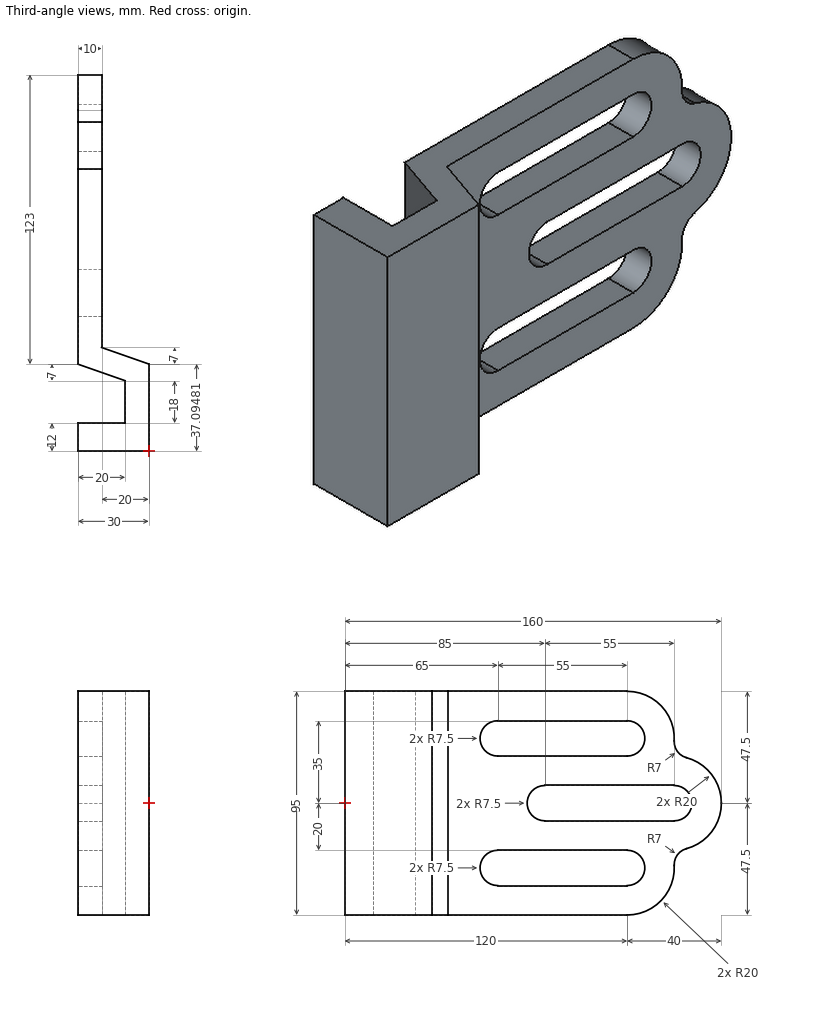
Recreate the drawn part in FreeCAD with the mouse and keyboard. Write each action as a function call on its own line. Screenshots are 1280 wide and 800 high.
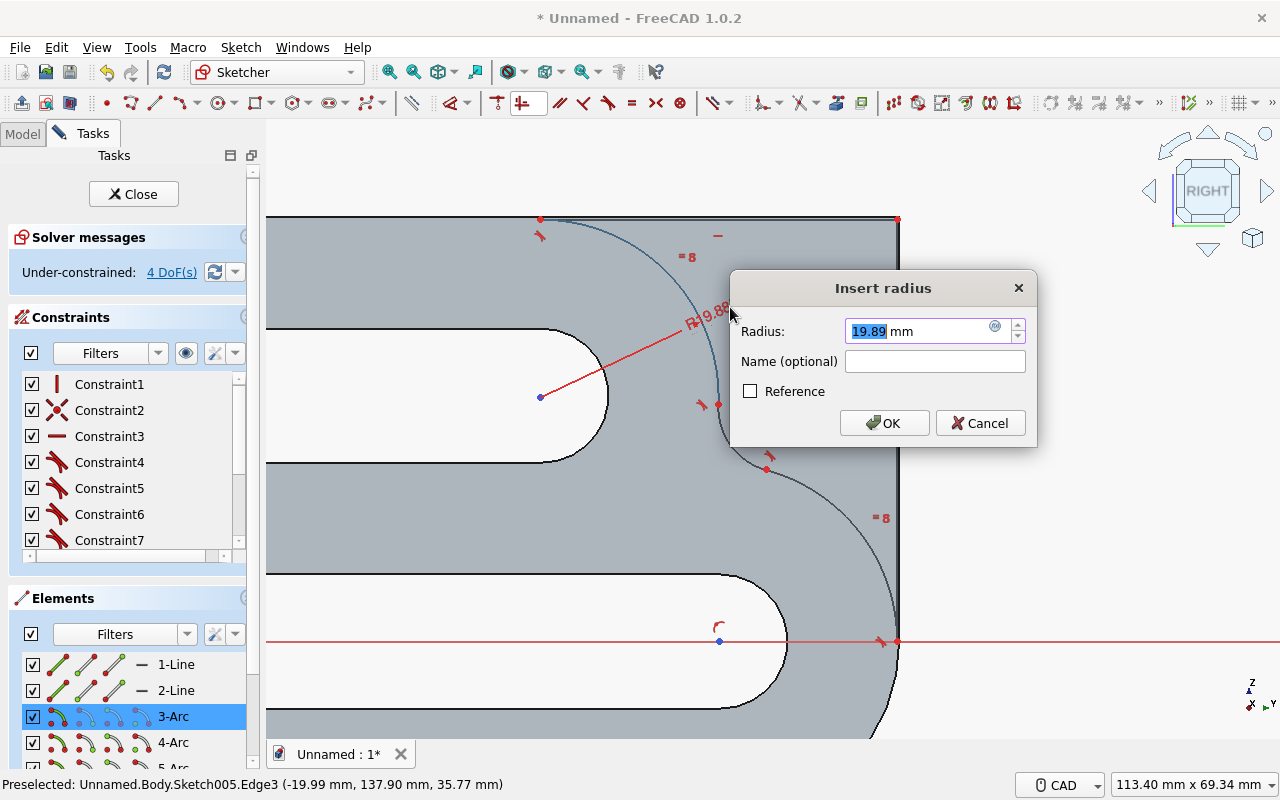
text(20)
key(Return)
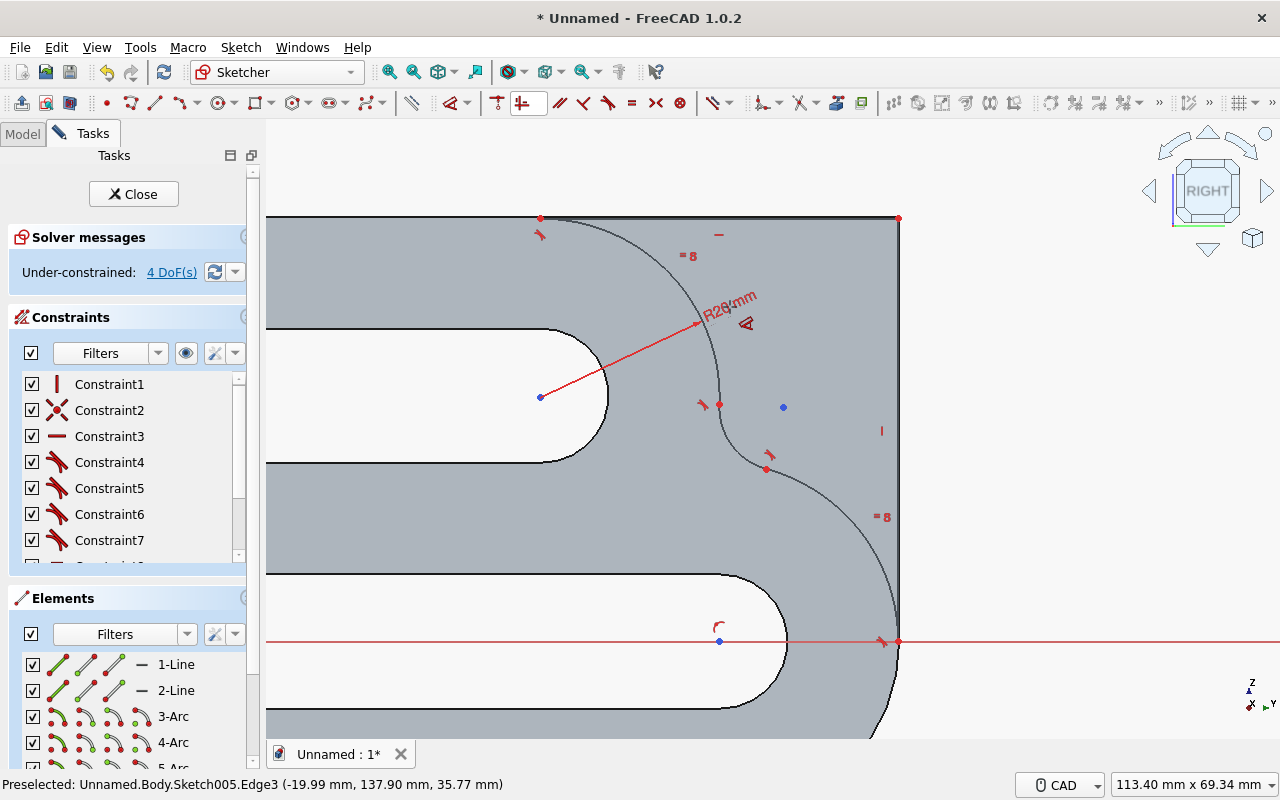
click(724, 430)
click(694, 441)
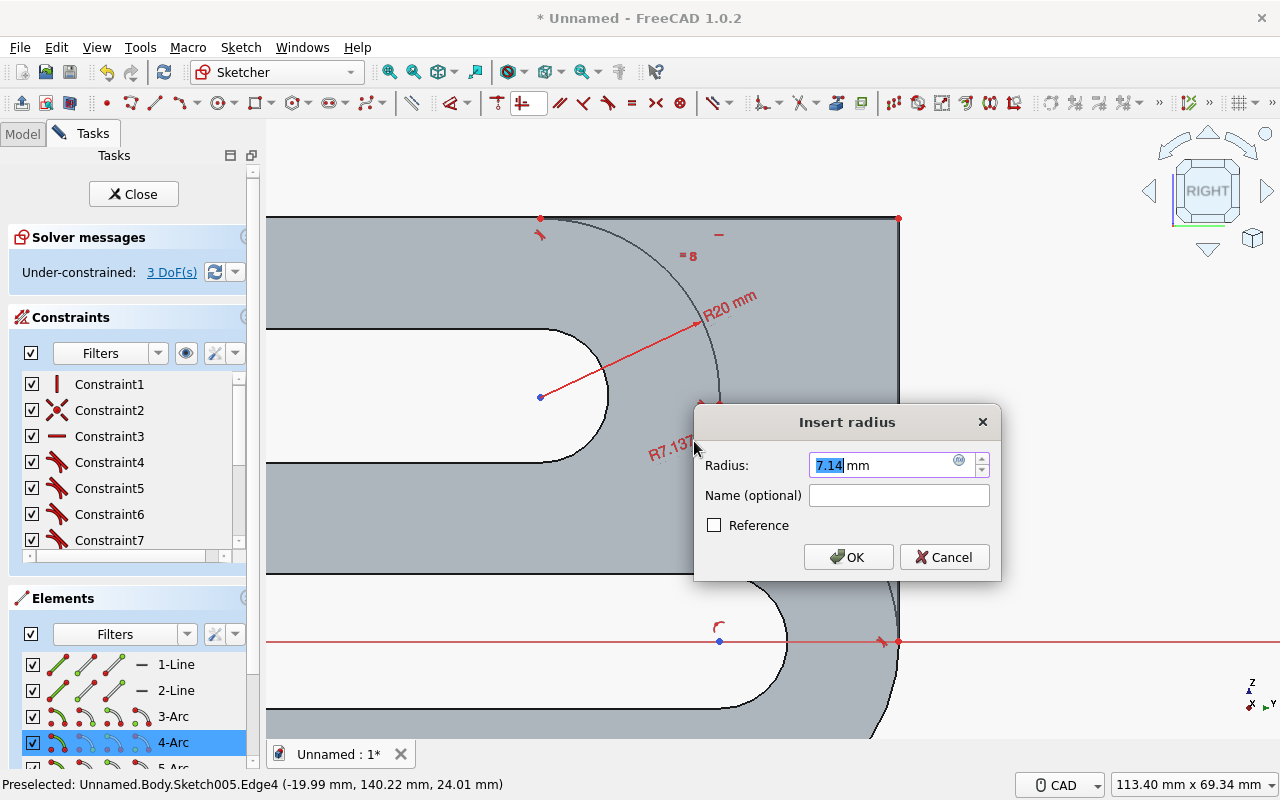
text(7)
key(Return)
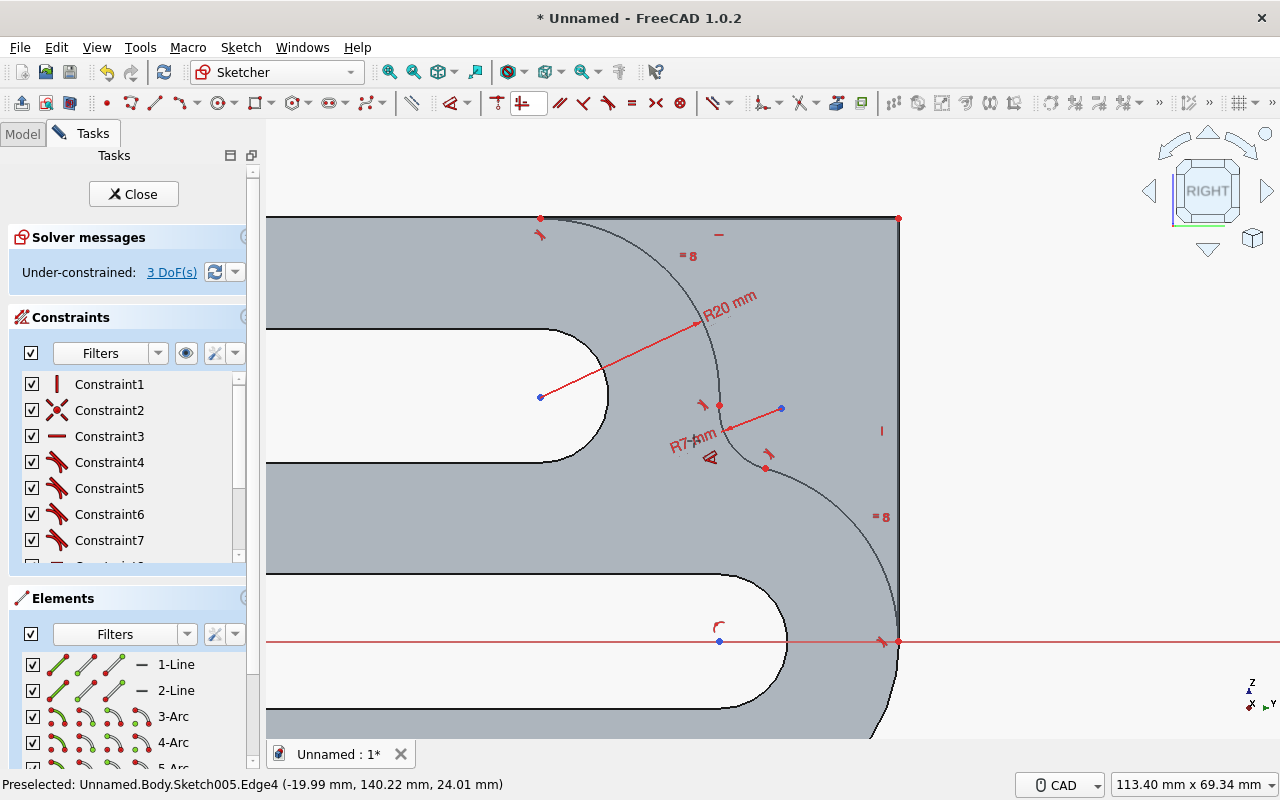
click(791, 219)
click(719, 185)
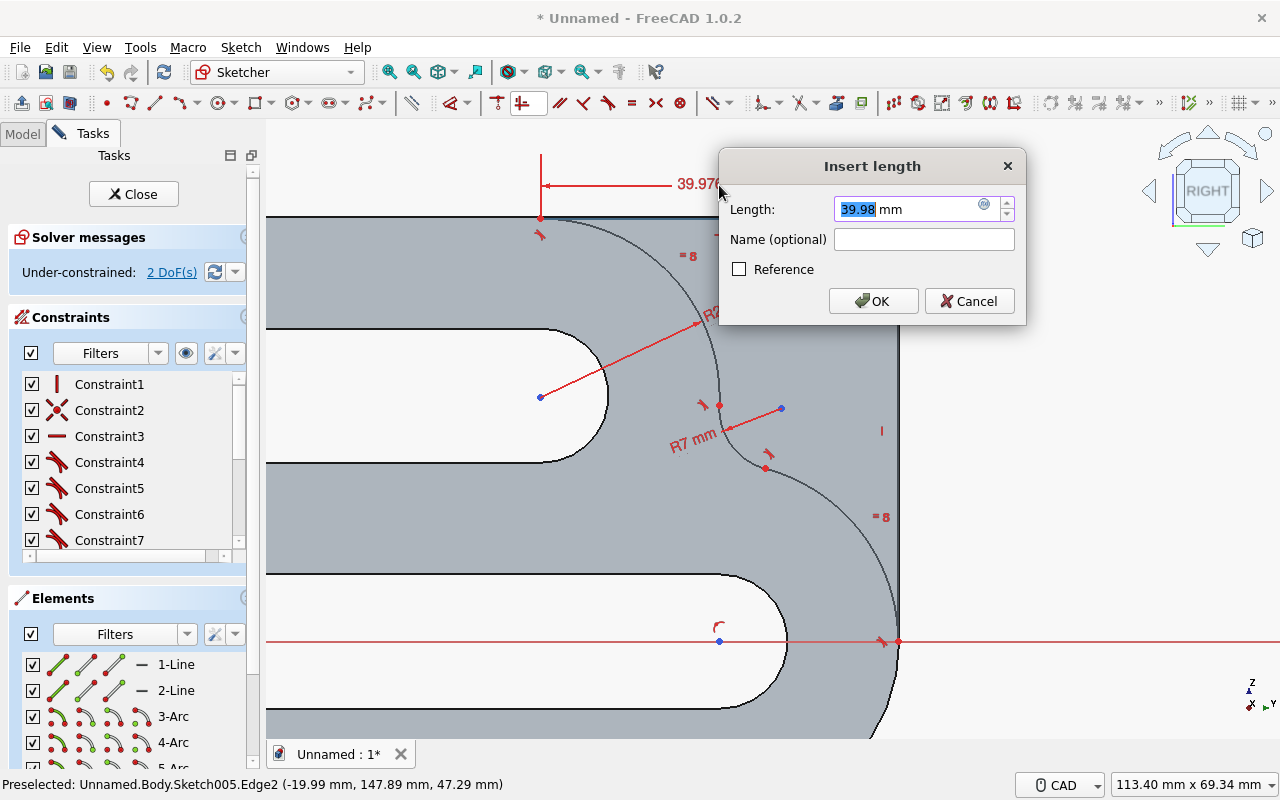
text(40)
key(Return)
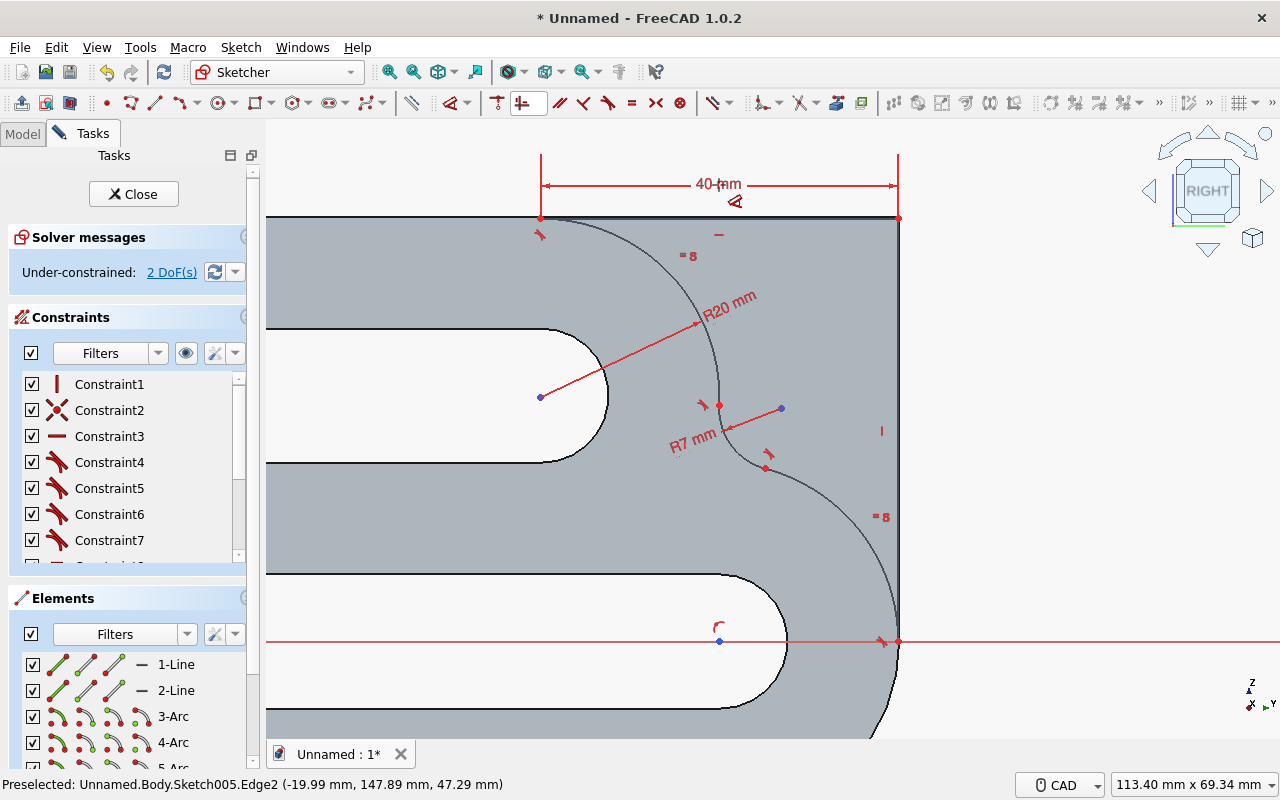
click(898, 515)
click(932, 430)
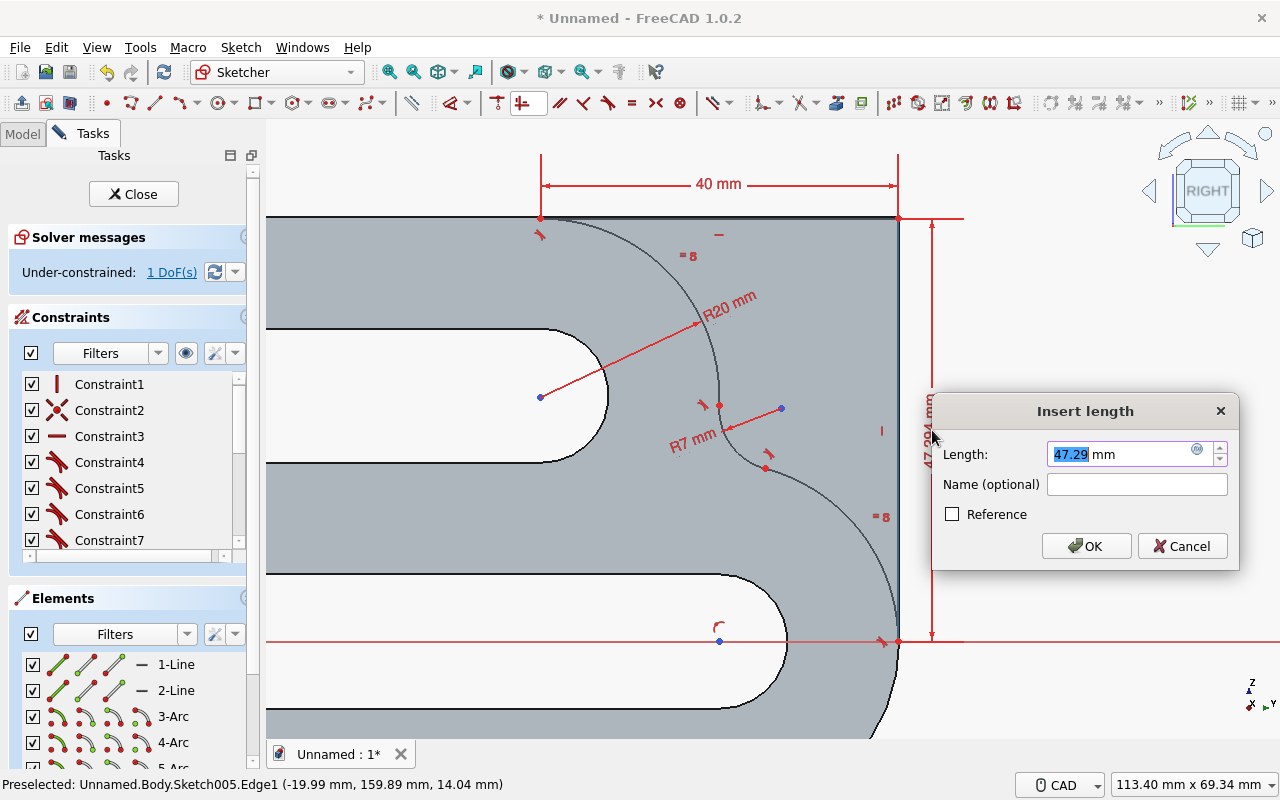
text(47.5)
key(Return)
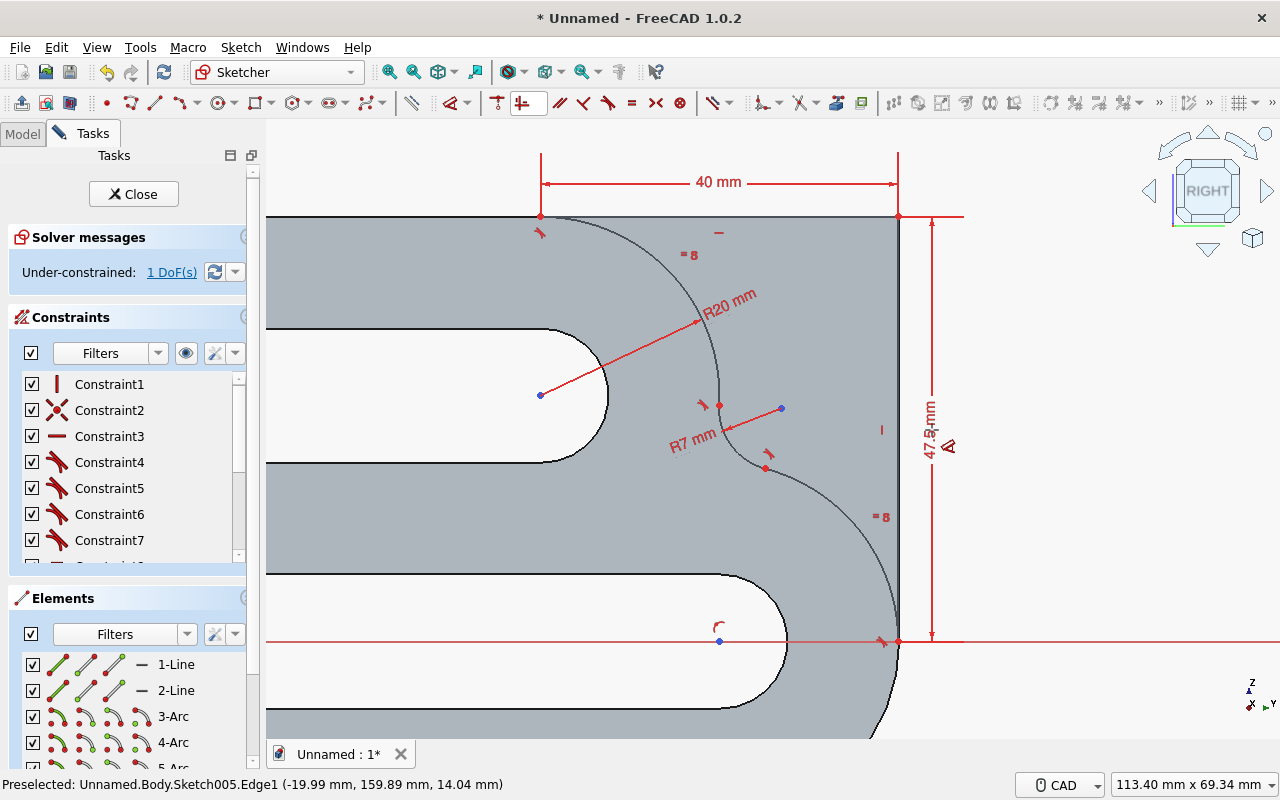
click(898, 642)
click(596, 676)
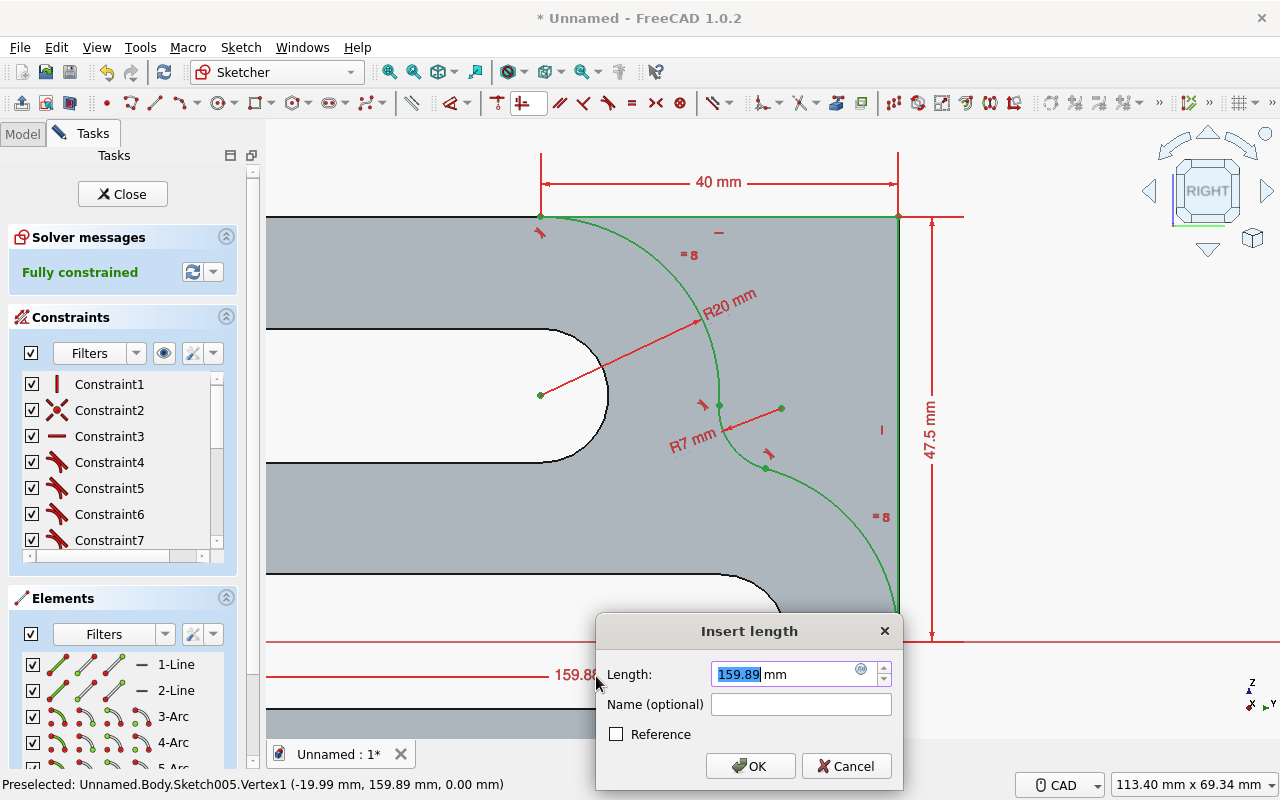
text(160)
key(Return)
key(Escape)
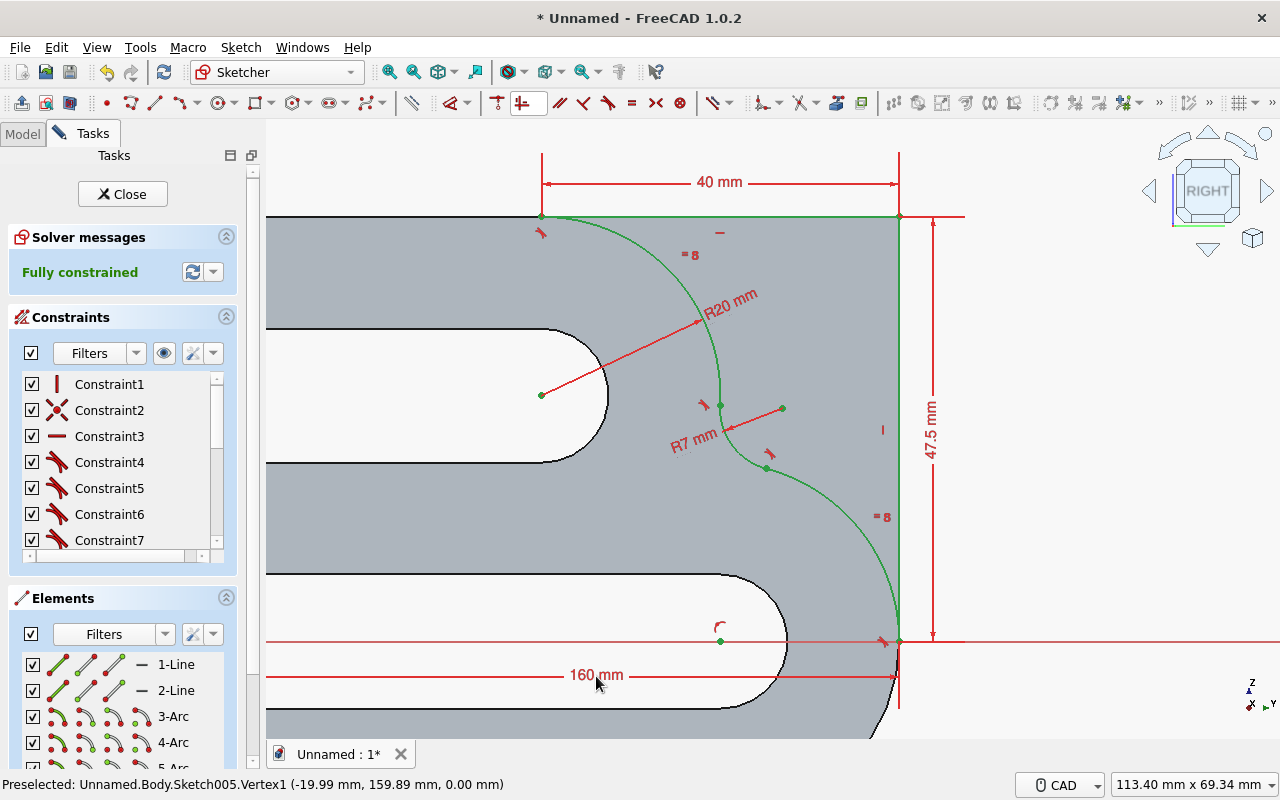
click(123, 194)